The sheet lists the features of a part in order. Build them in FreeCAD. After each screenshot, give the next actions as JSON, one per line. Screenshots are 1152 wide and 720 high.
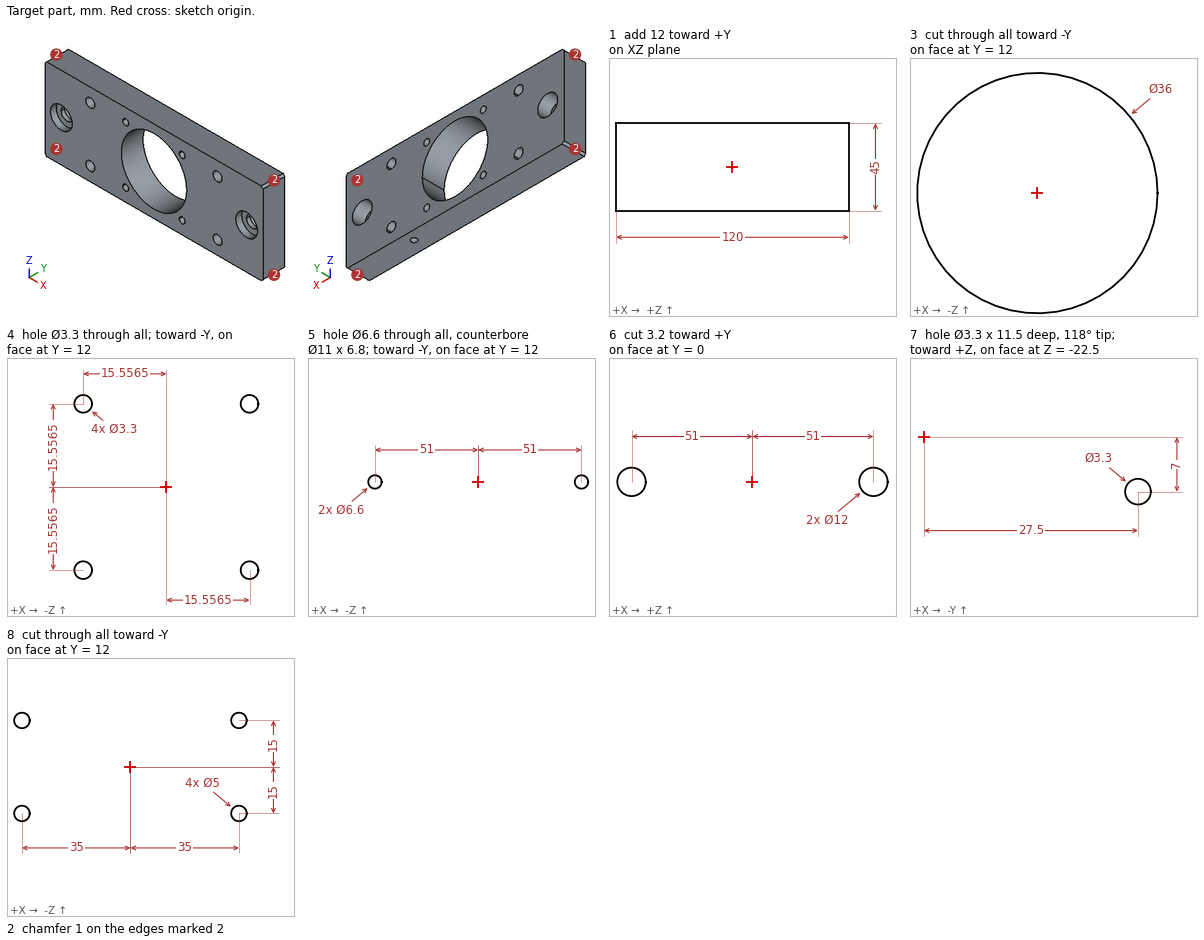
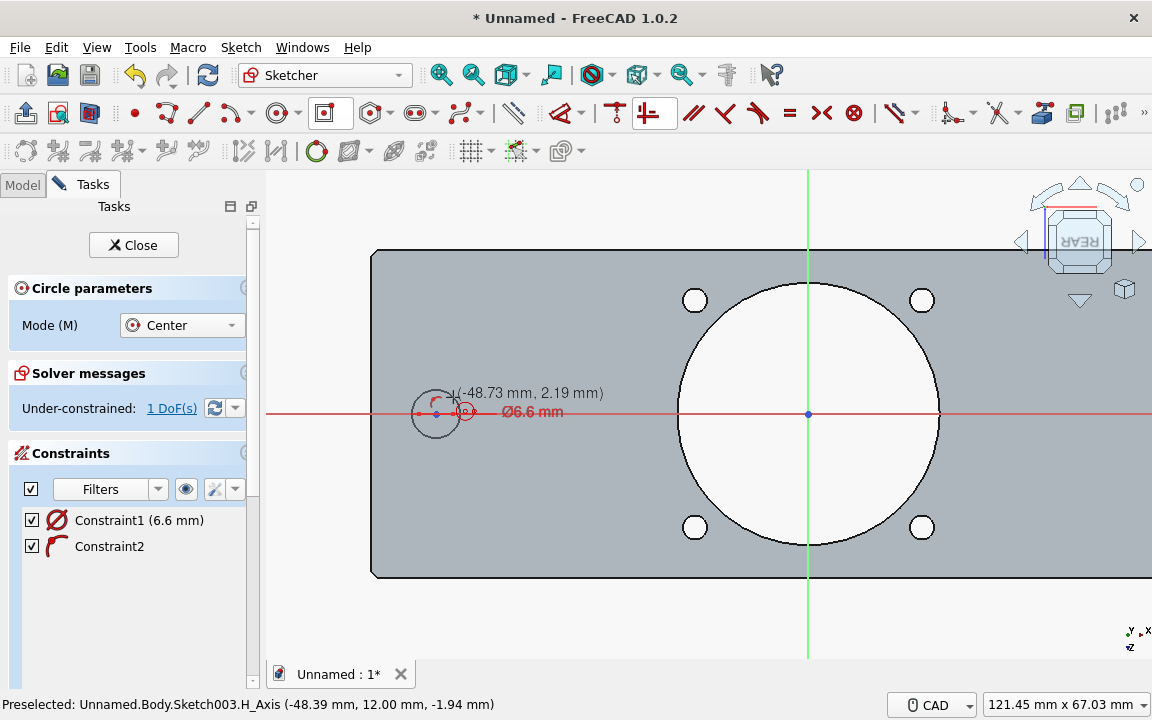
{"action": "scroll", "coordinate": [299, 416], "scroll_direction": "down", "scroll_amount": 2}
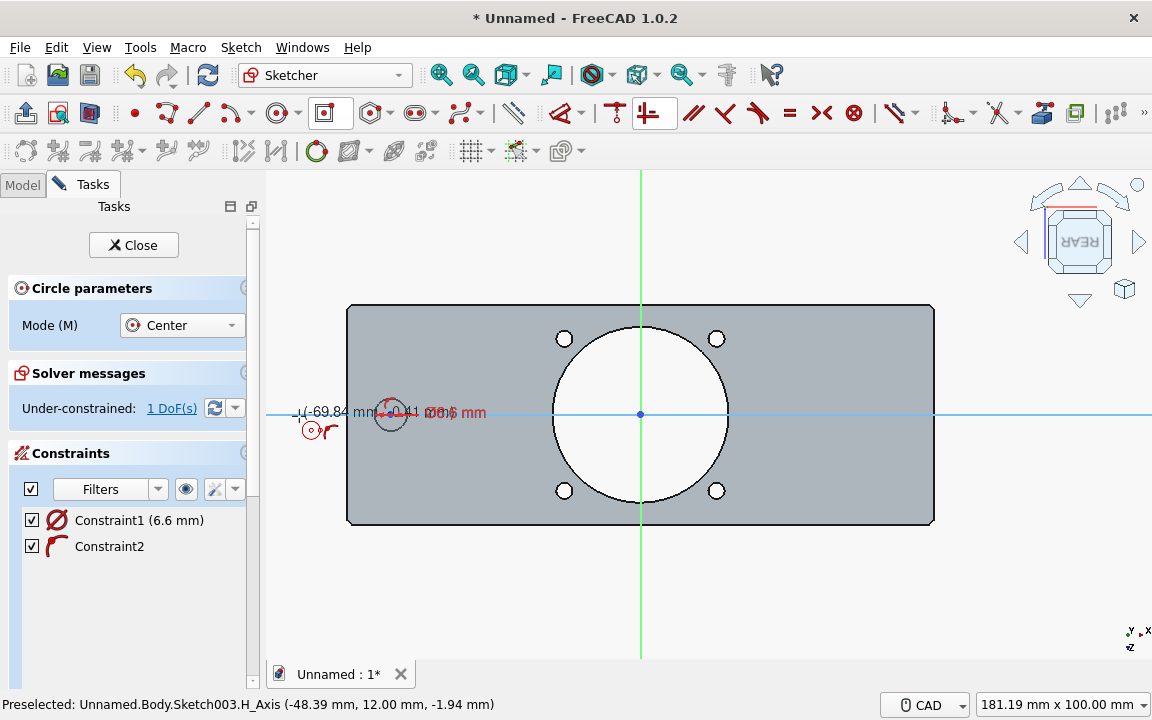
{"action": "scroll", "coordinate": [890, 415], "scroll_direction": "up", "scroll_amount": 2}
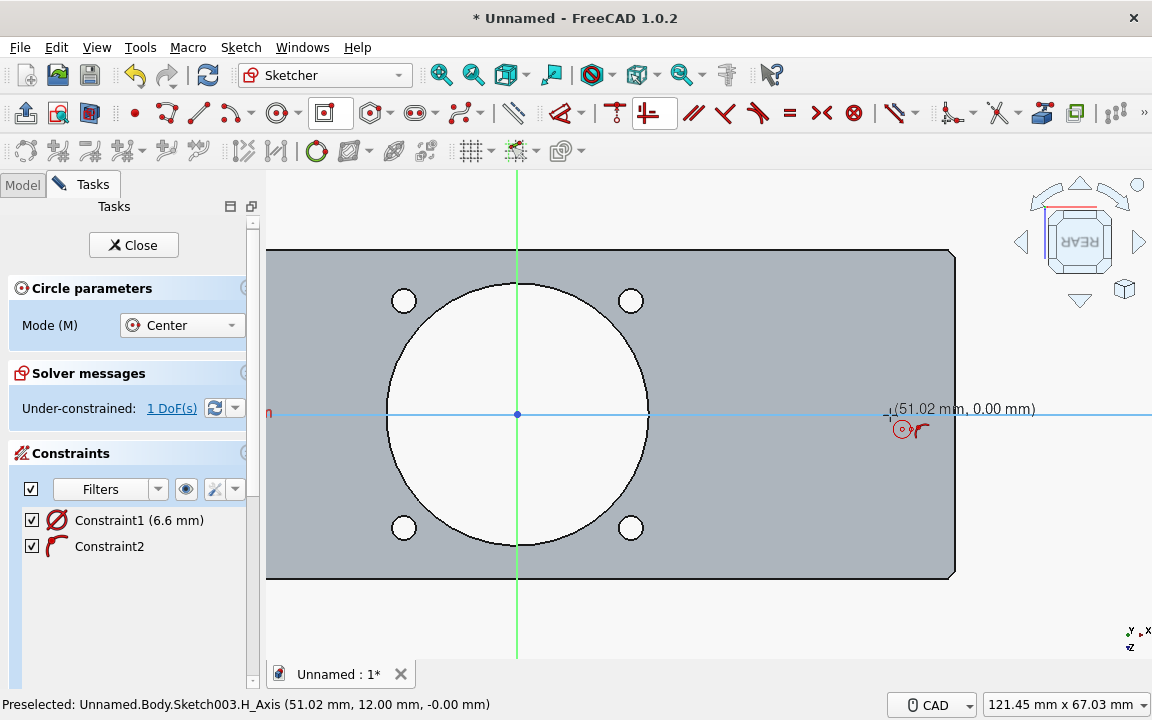
{"action": "left_click", "coordinate": [890, 414]}
{"action": "mouse_move", "coordinate": [907, 397]}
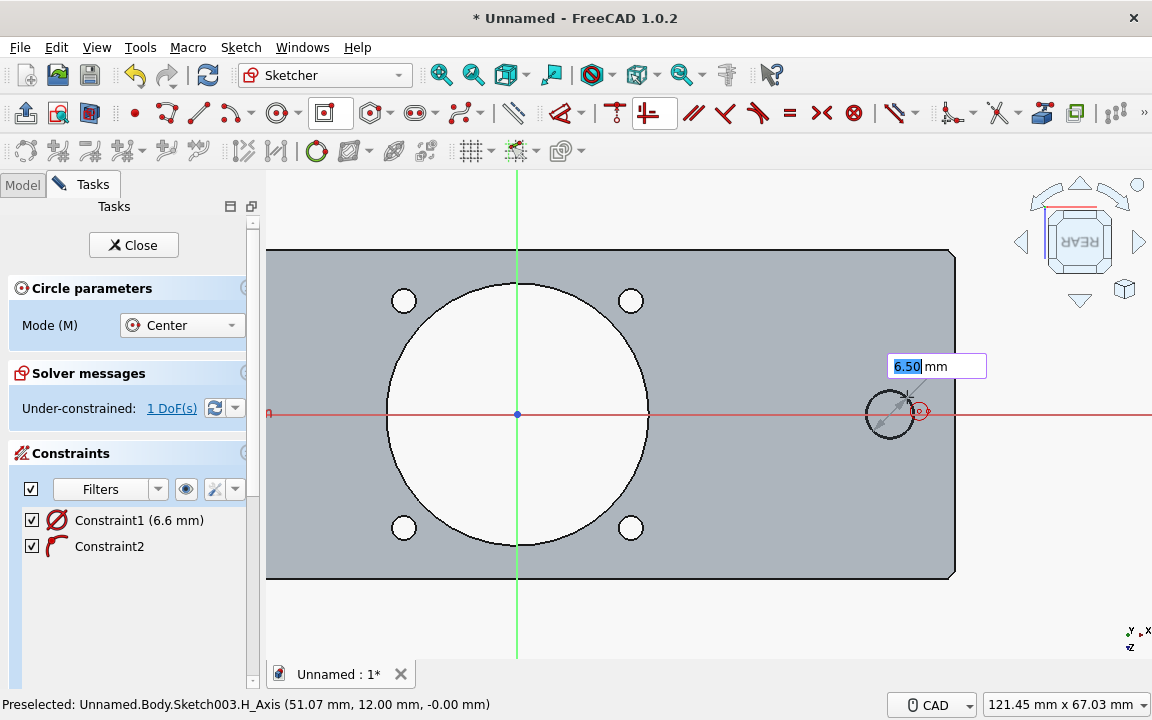
{"action": "type", "text": "6.6"}
{"action": "key", "text": "Return"}
{"action": "key", "text": "Escape"}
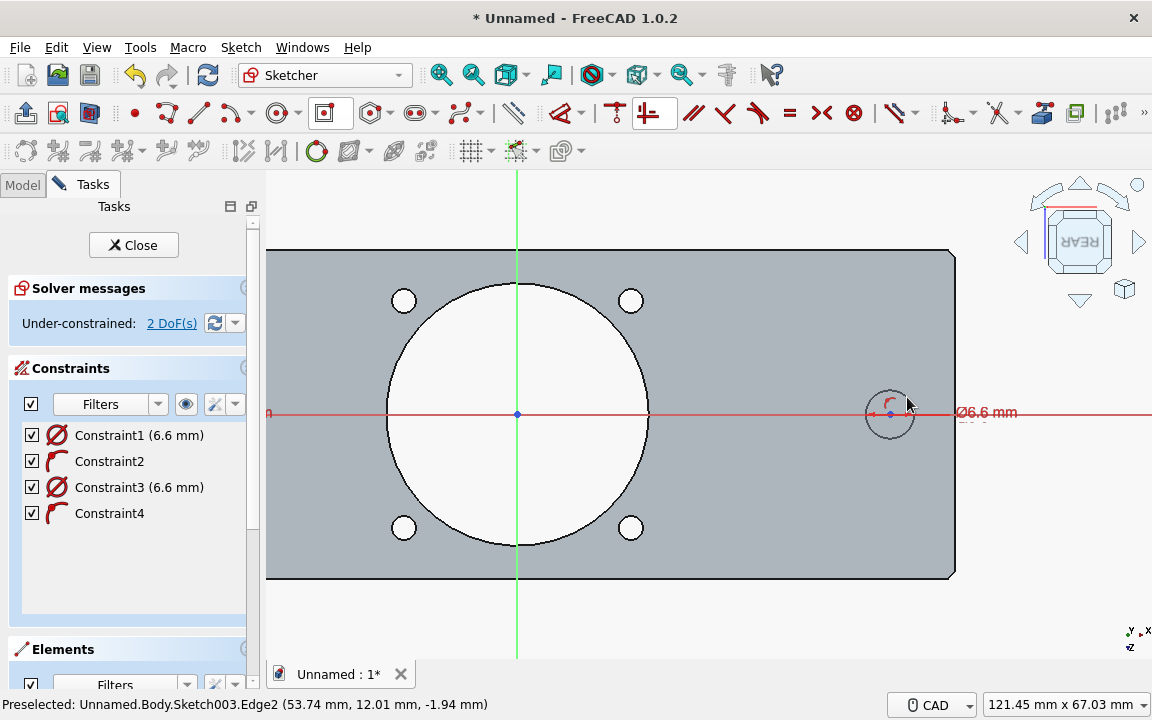
{"action": "left_click", "coordinate": [560, 114]}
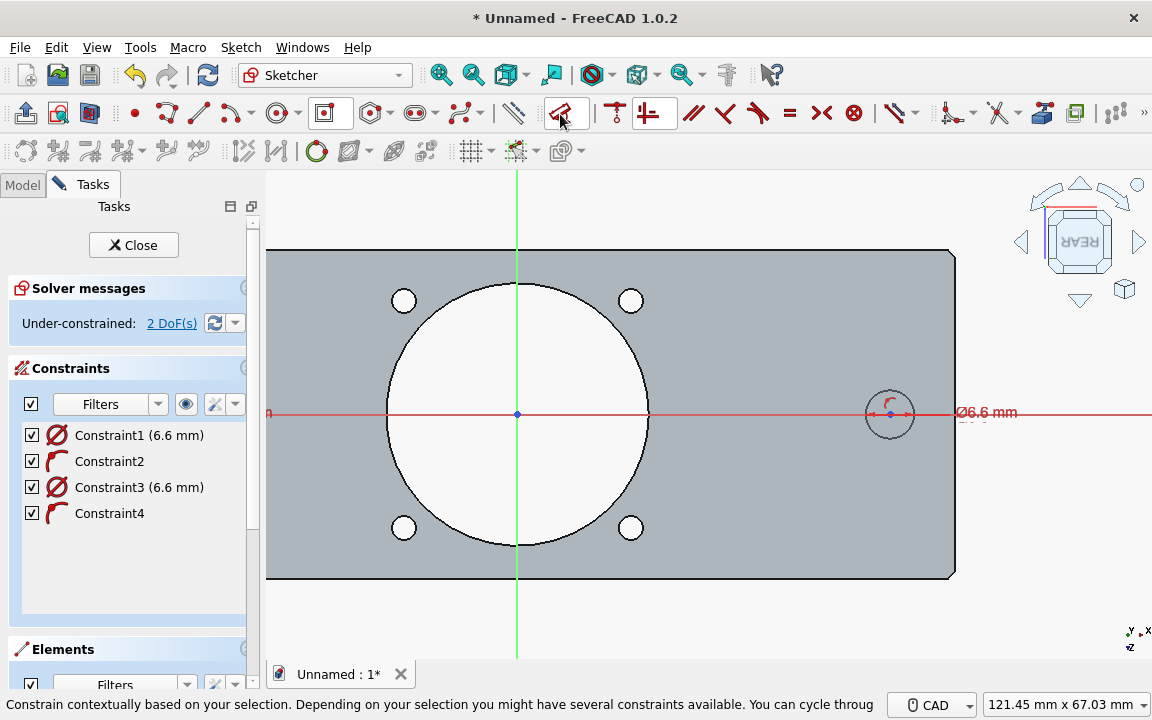
{"action": "scroll", "coordinate": [891, 415], "scroll_direction": "down", "scroll_amount": 2}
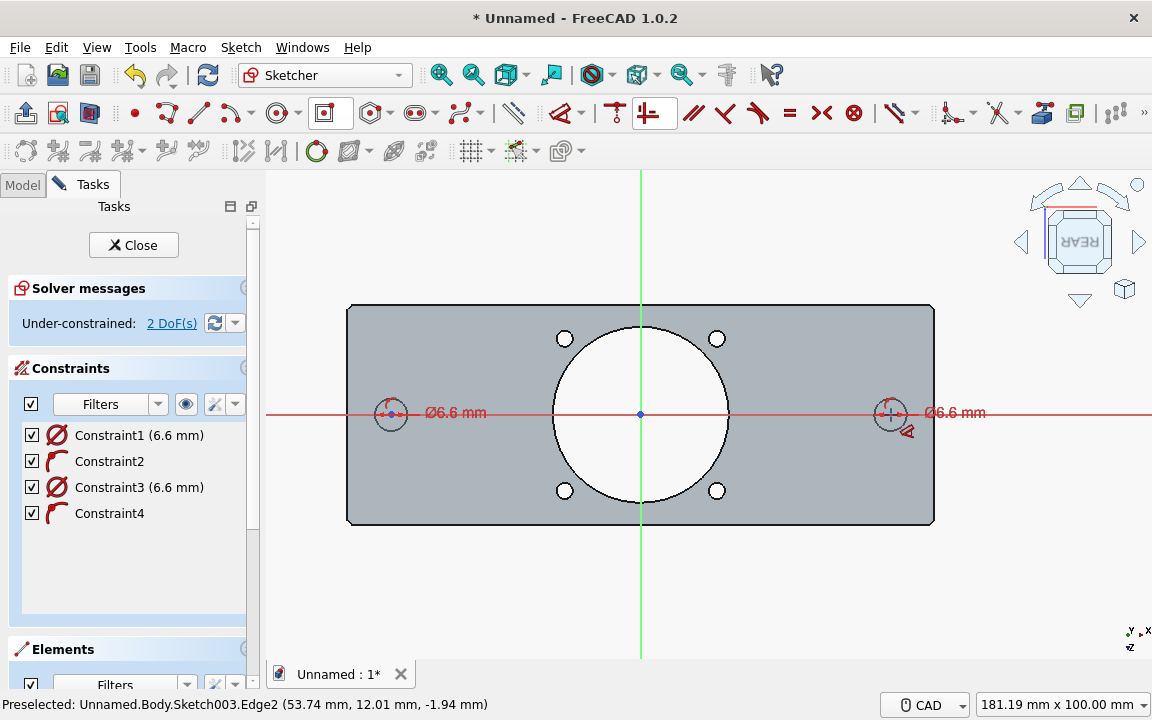
{"action": "left_click", "coordinate": [391, 415]}
{"action": "left_click", "coordinate": [516, 449]}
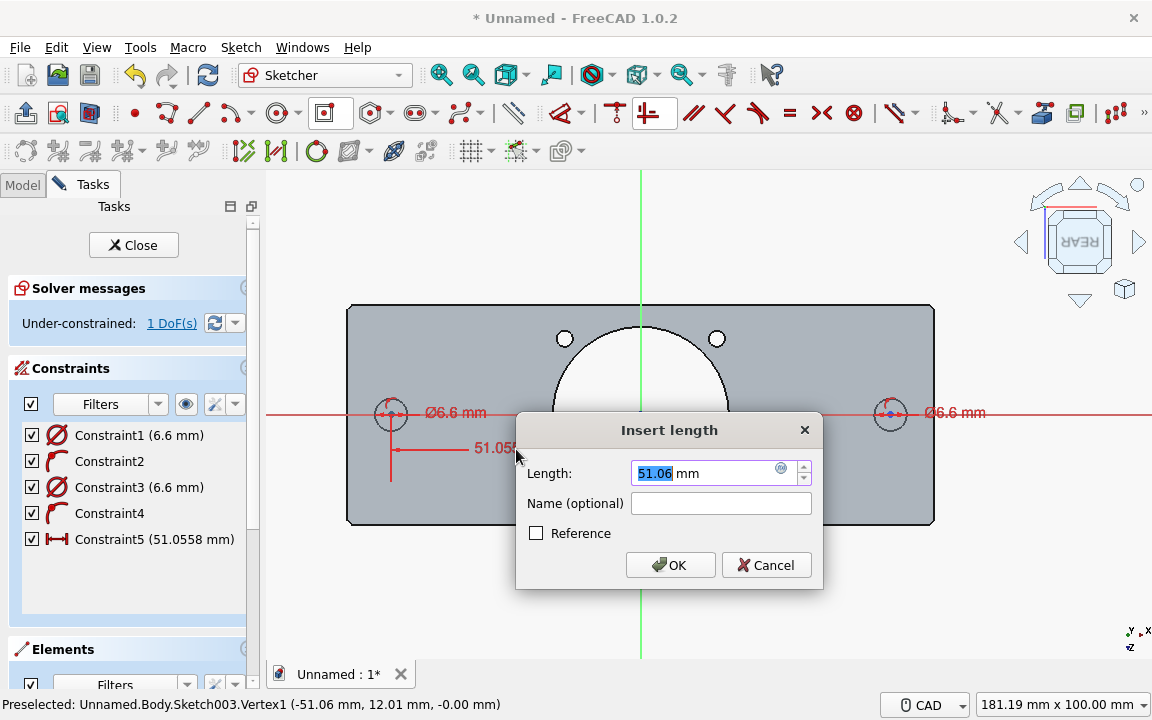
{"action": "type", "text": "51"}
{"action": "key", "text": "Return"}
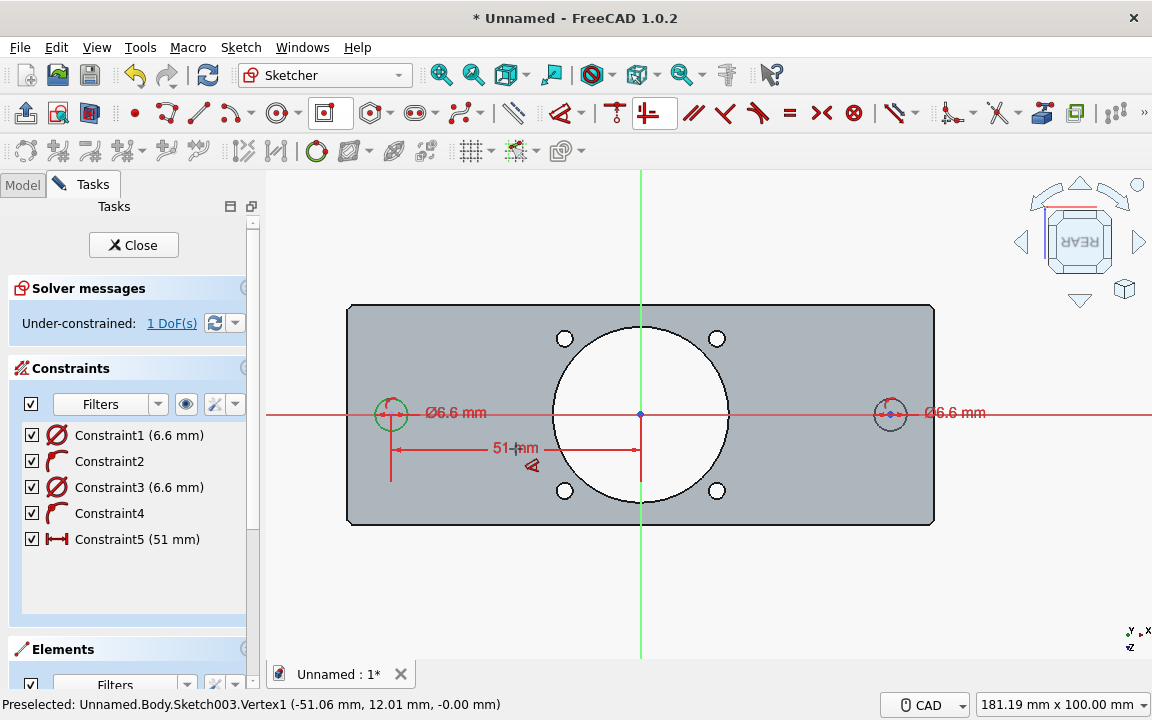
{"action": "left_click", "coordinate": [891, 415]}
{"action": "left_click", "coordinate": [766, 449]}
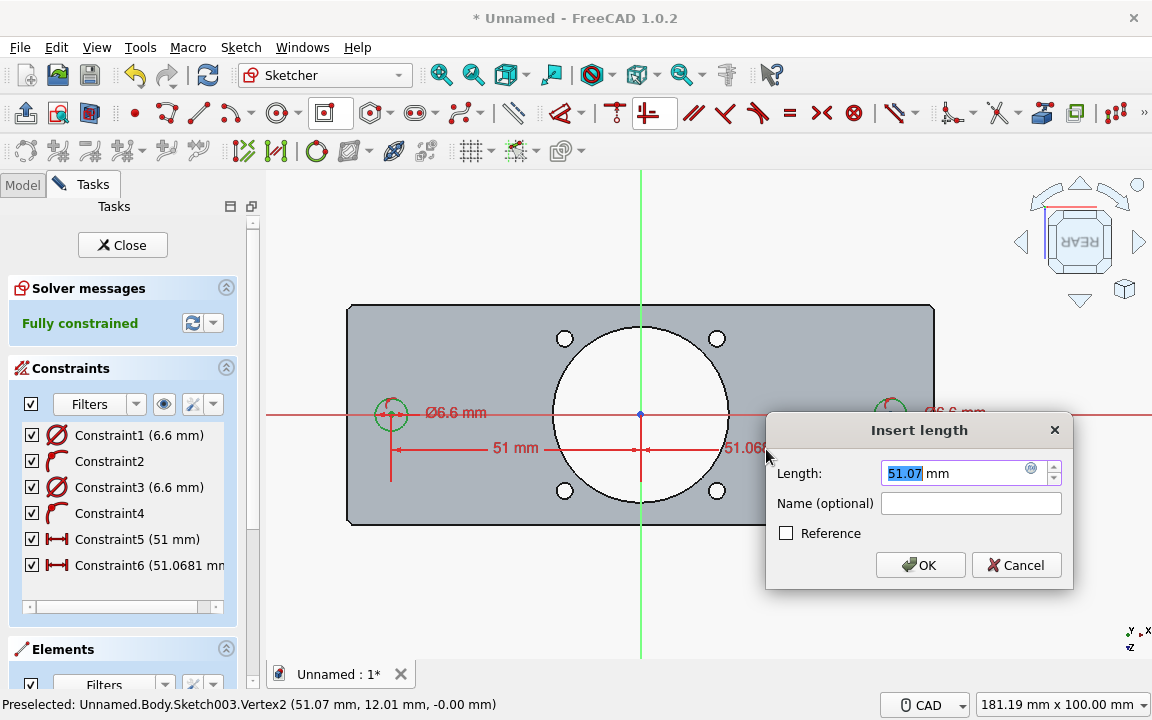
{"action": "type", "text": "51"}
{"action": "key", "text": "Return"}
{"action": "key", "text": "Escape"}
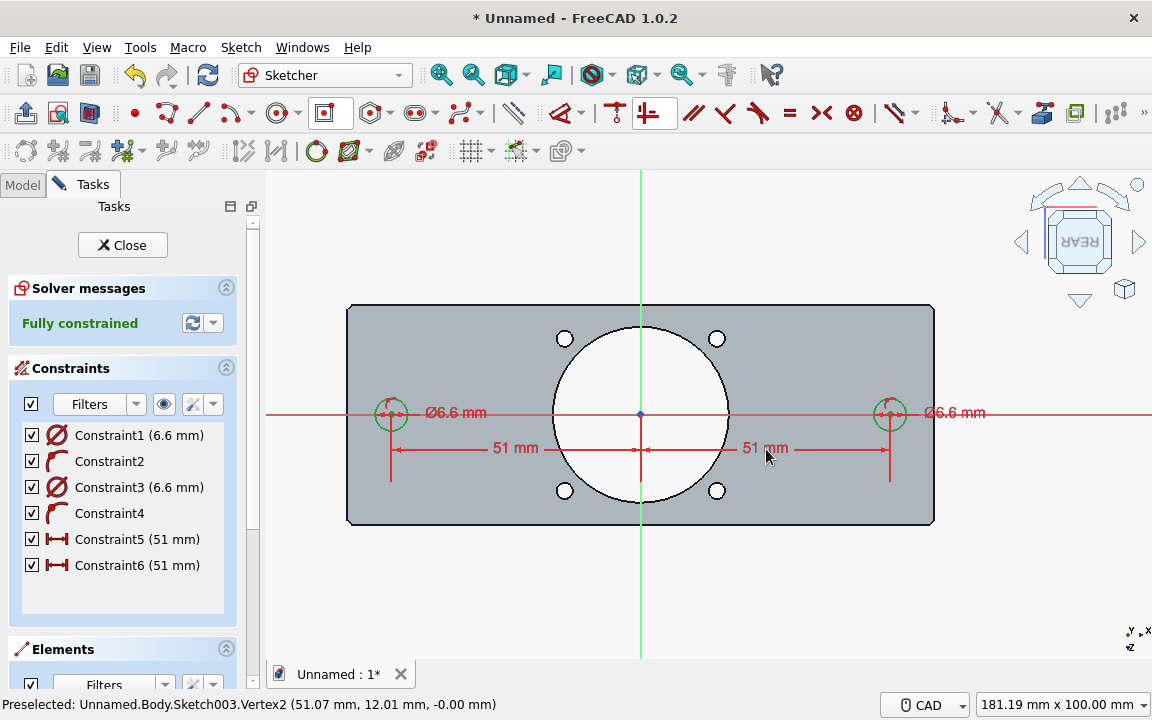
{"action": "left_click", "coordinate": [123, 245]}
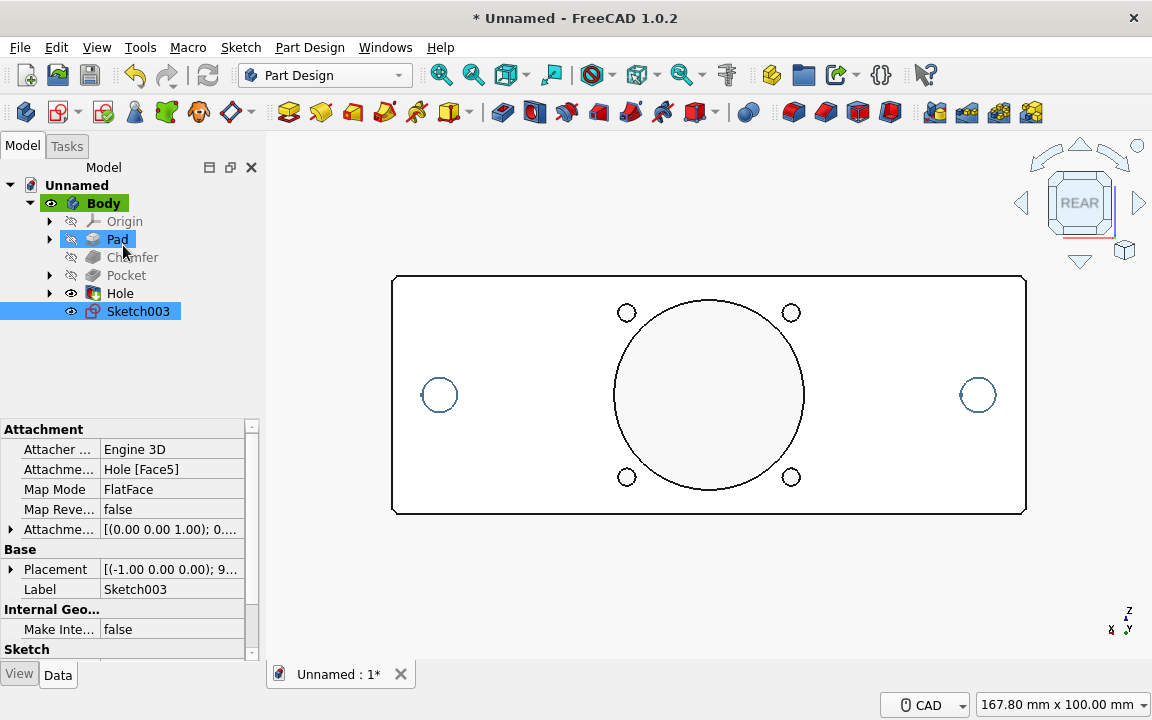
{"action": "left_click", "coordinate": [536, 112]}